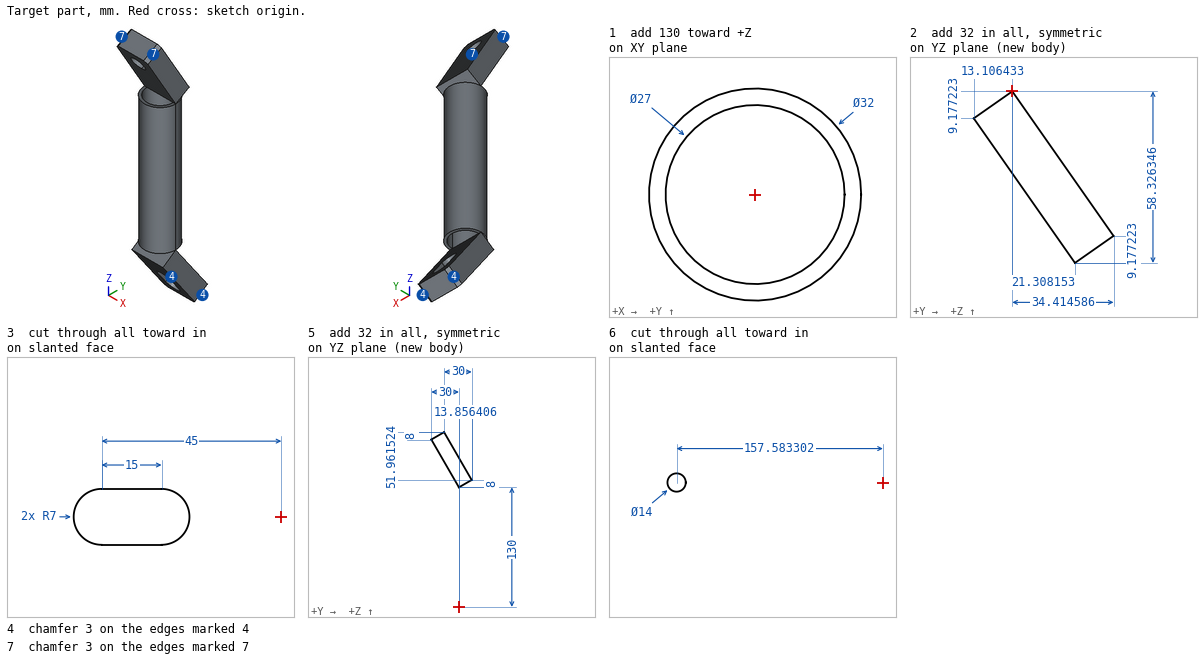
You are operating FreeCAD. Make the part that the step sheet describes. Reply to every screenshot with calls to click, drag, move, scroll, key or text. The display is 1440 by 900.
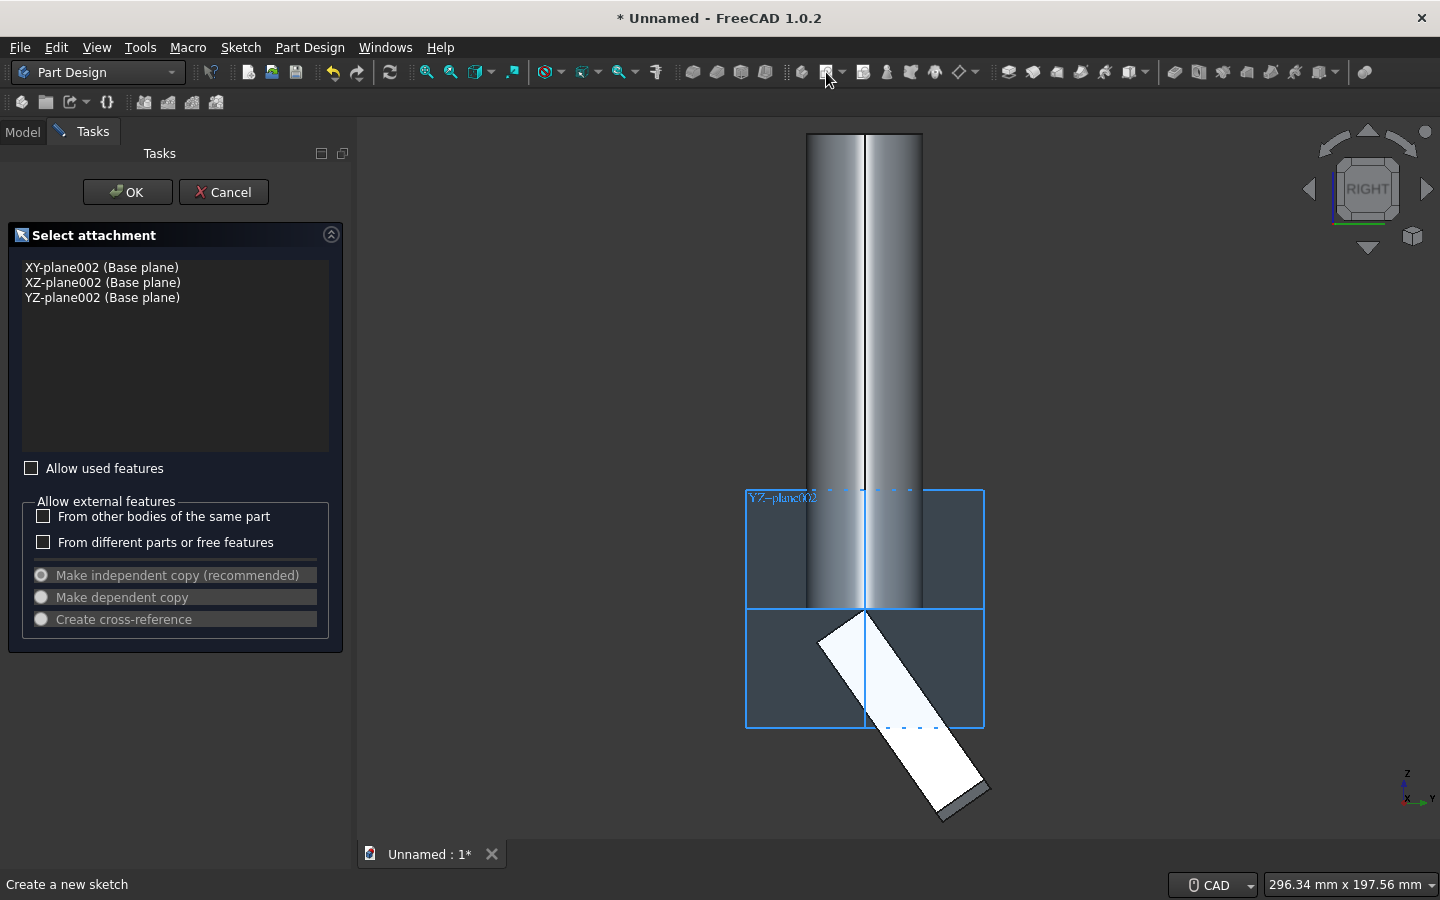
click(82, 298)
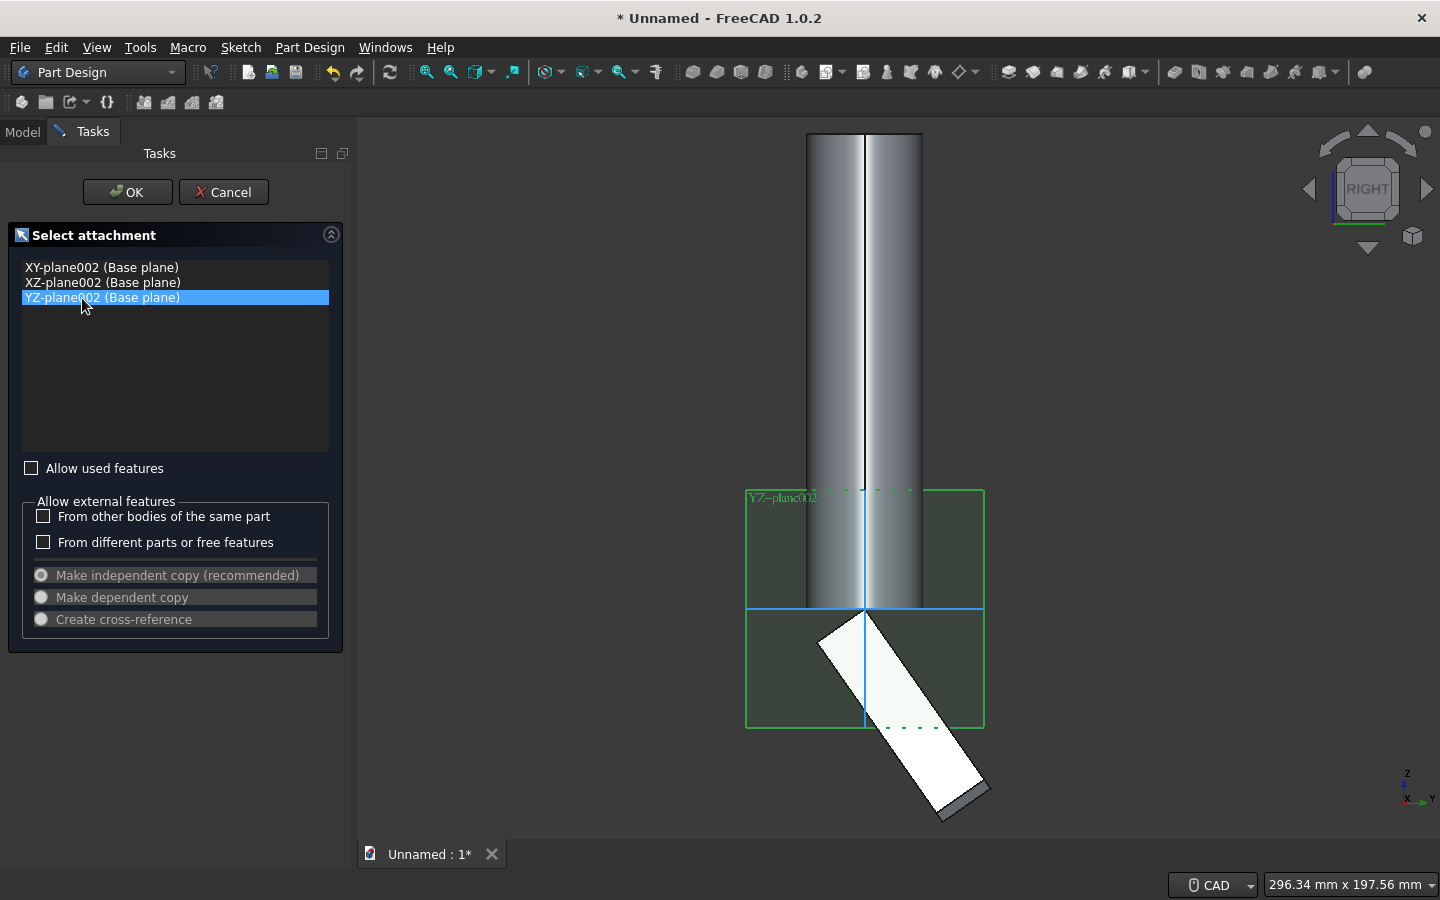
click(128, 192)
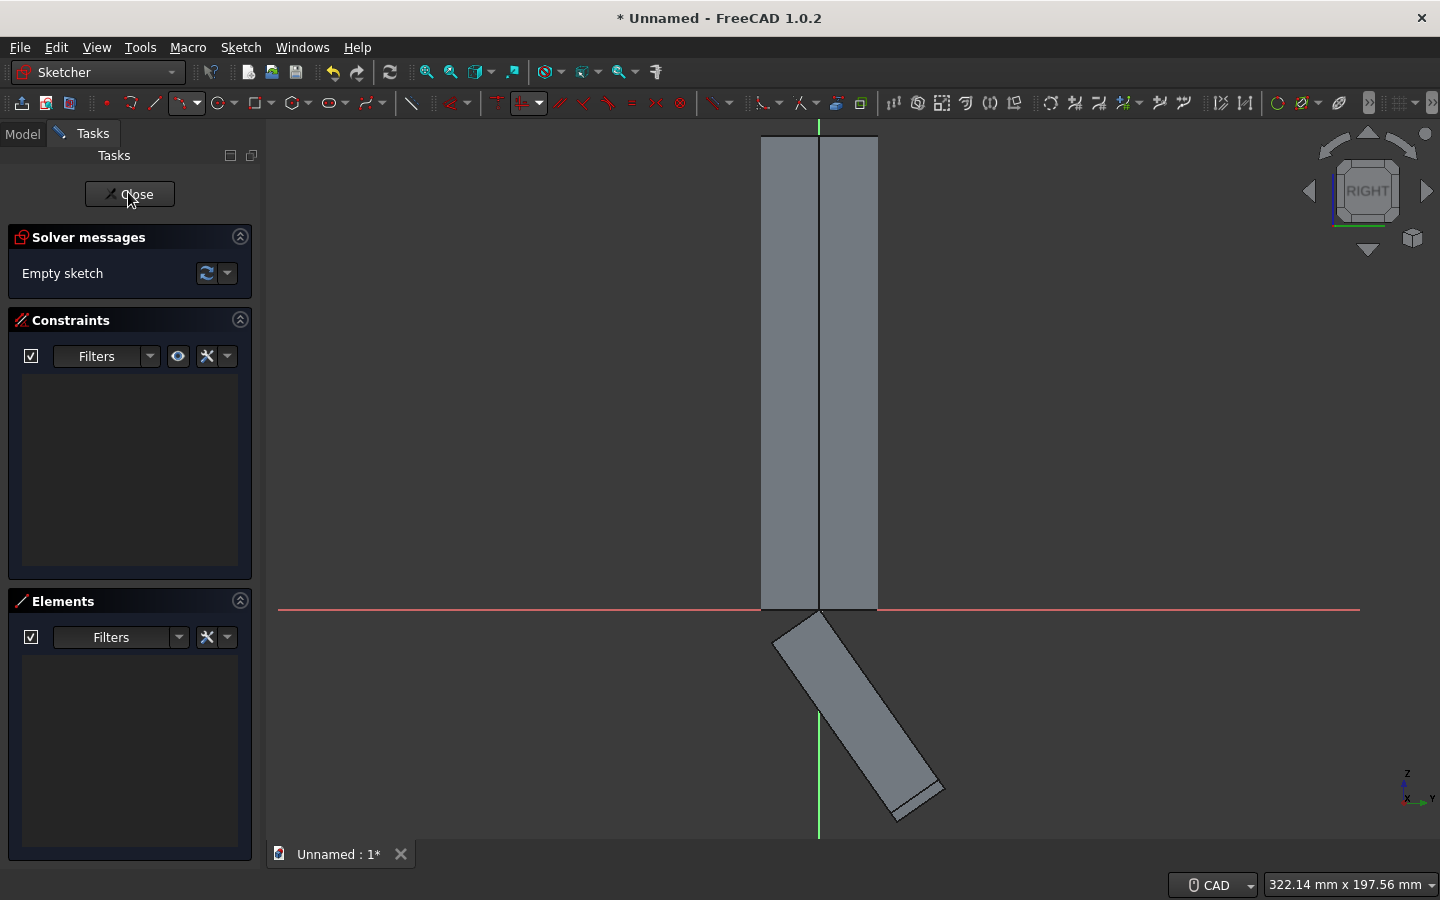
scroll(784, 479, down, 5)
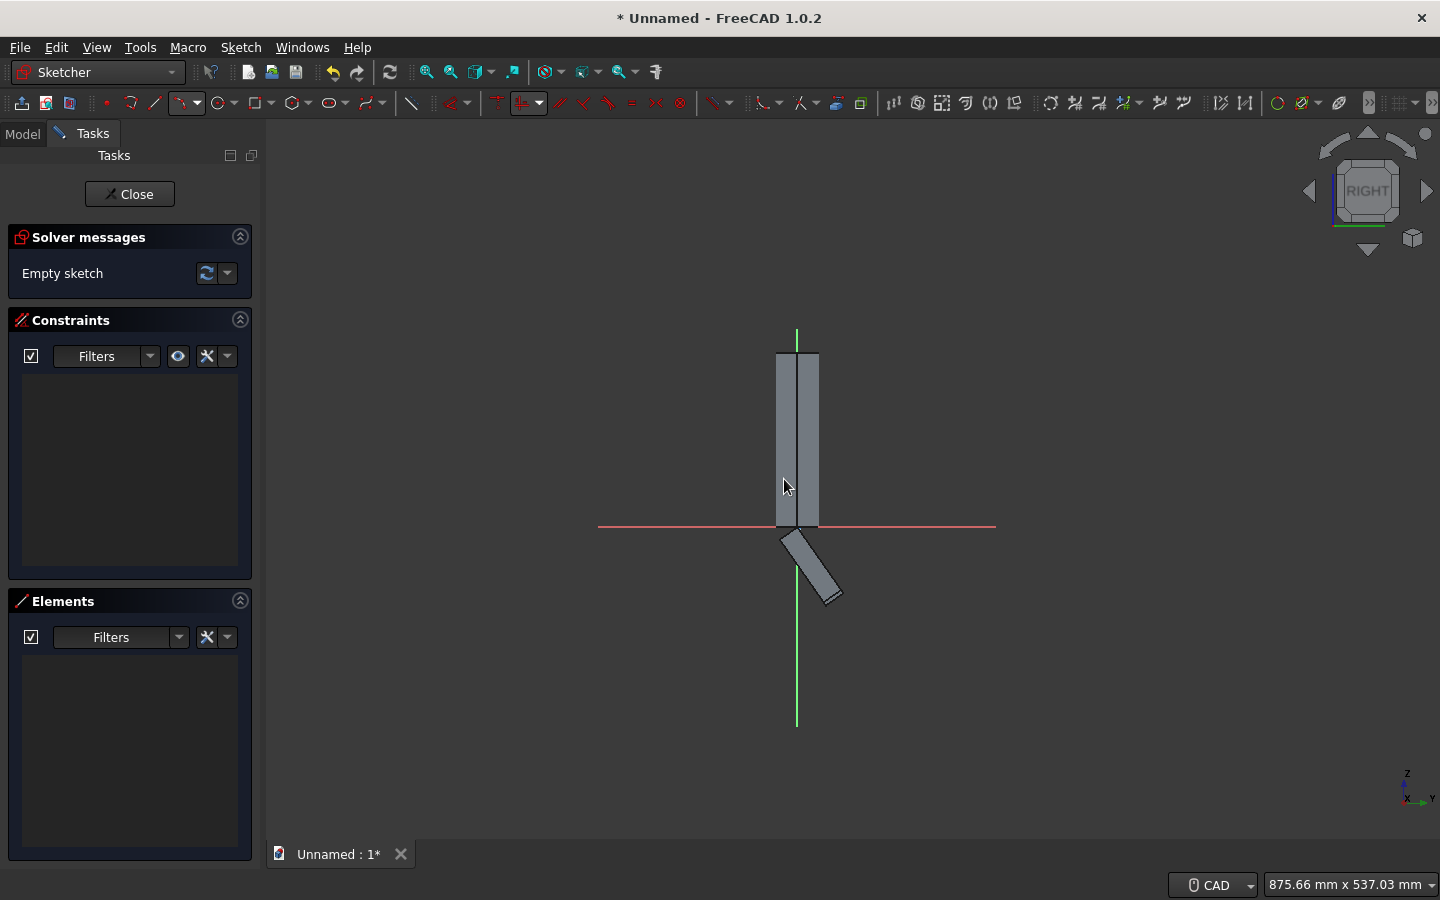
scroll(787, 280, up, 9)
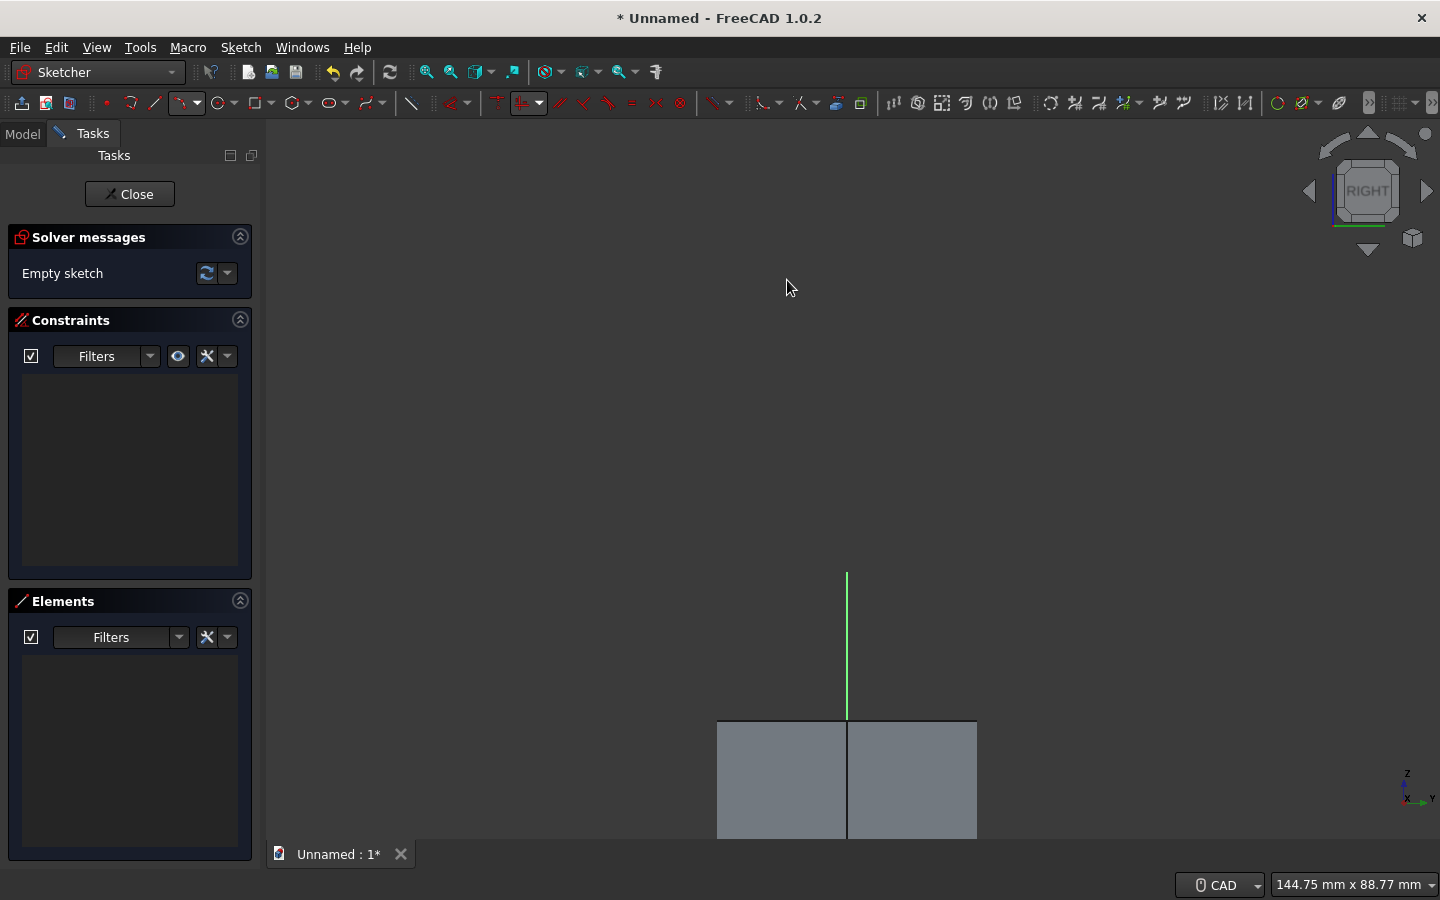
key(g)
key(m)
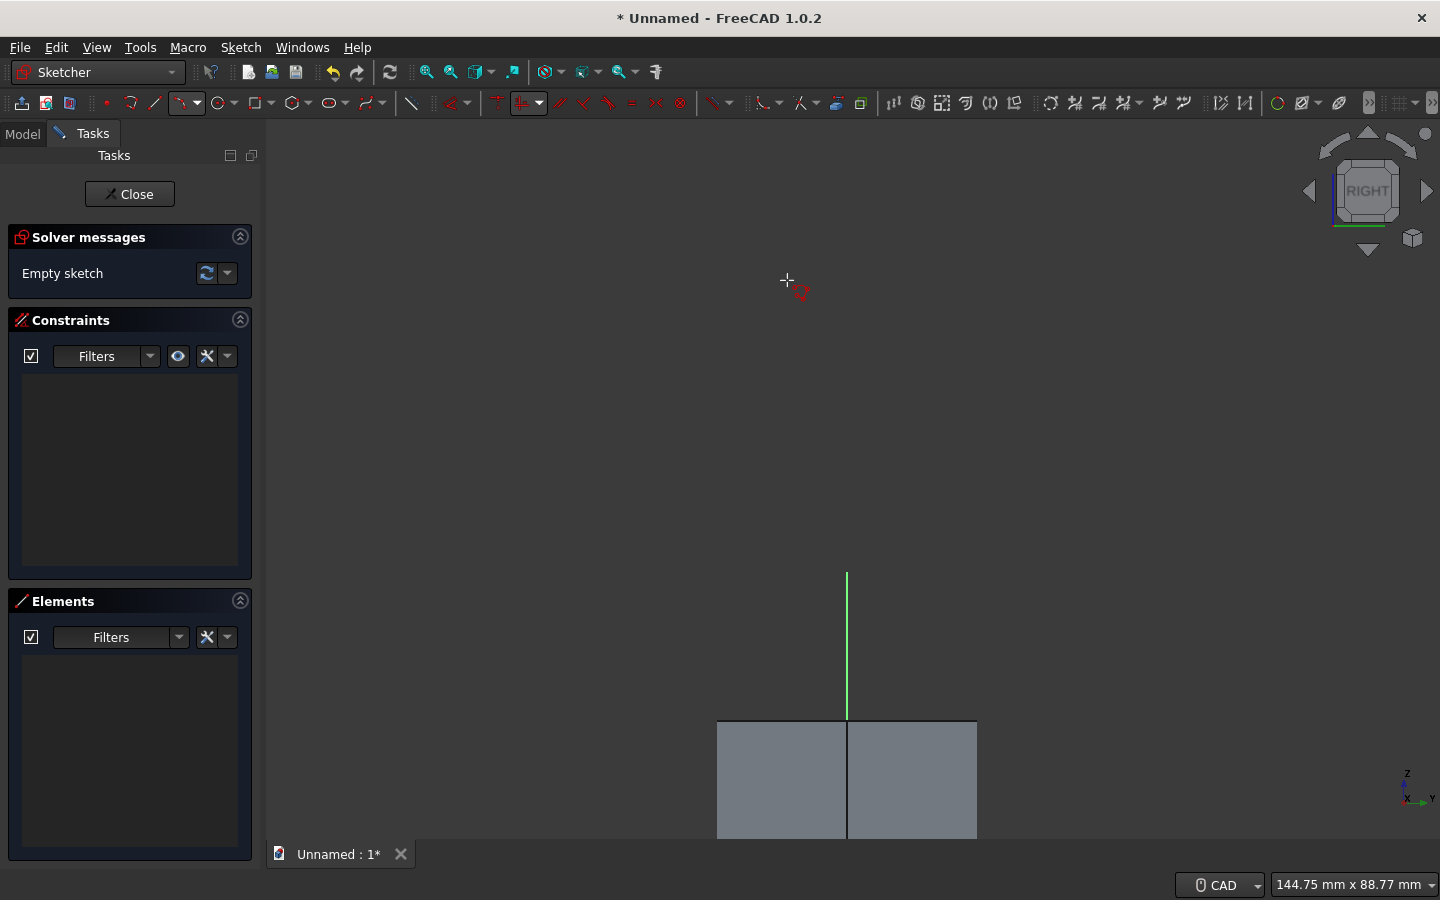
click(847, 721)
click(960, 656)
click(716, 235)
click(604, 299)
click(847, 722)
key(Escape)
key(Escape)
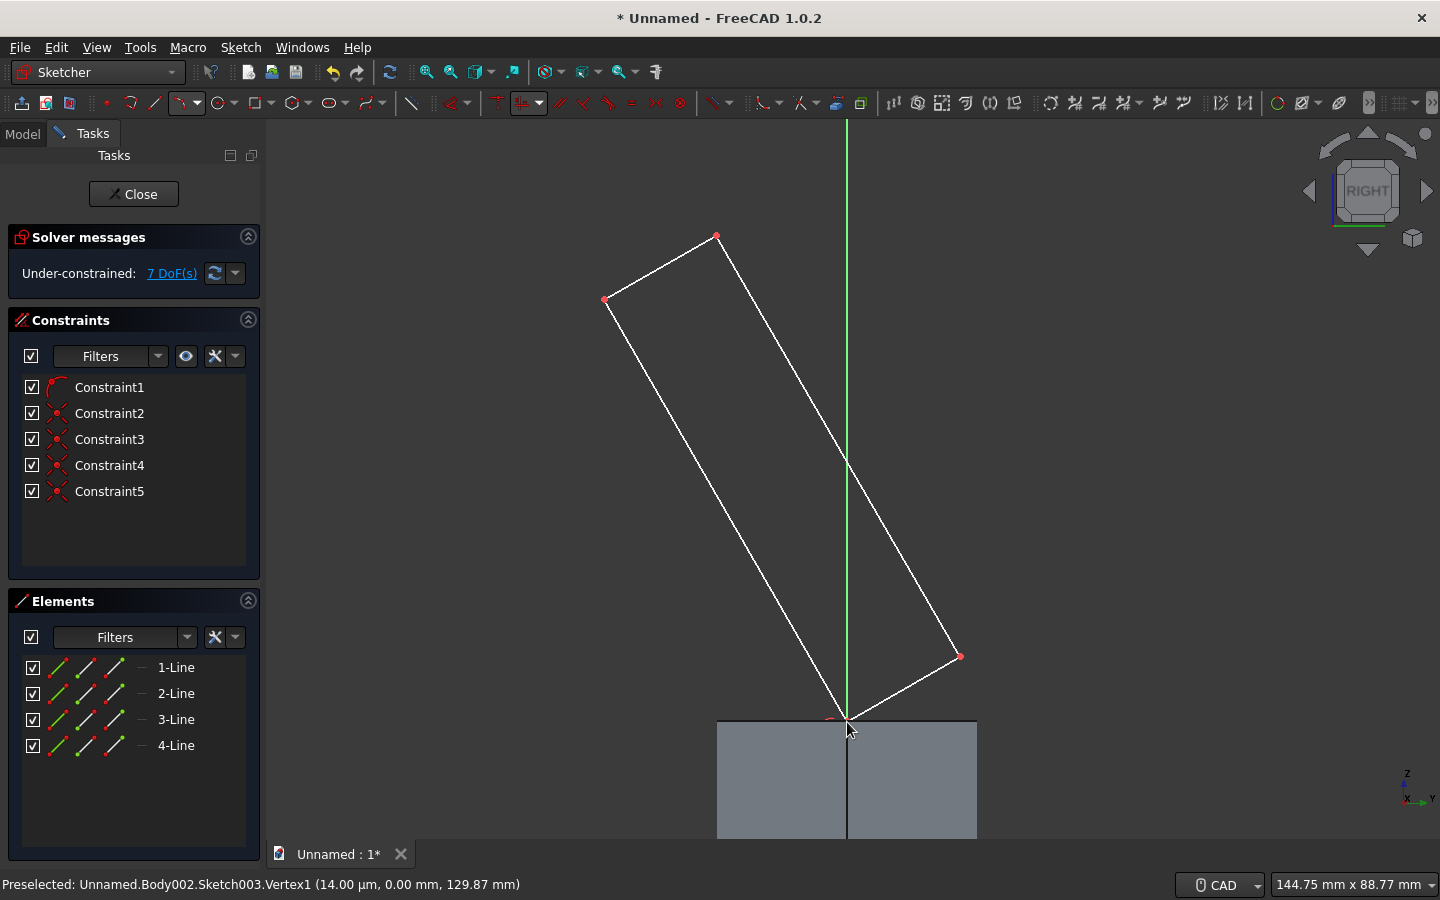
click(450, 104)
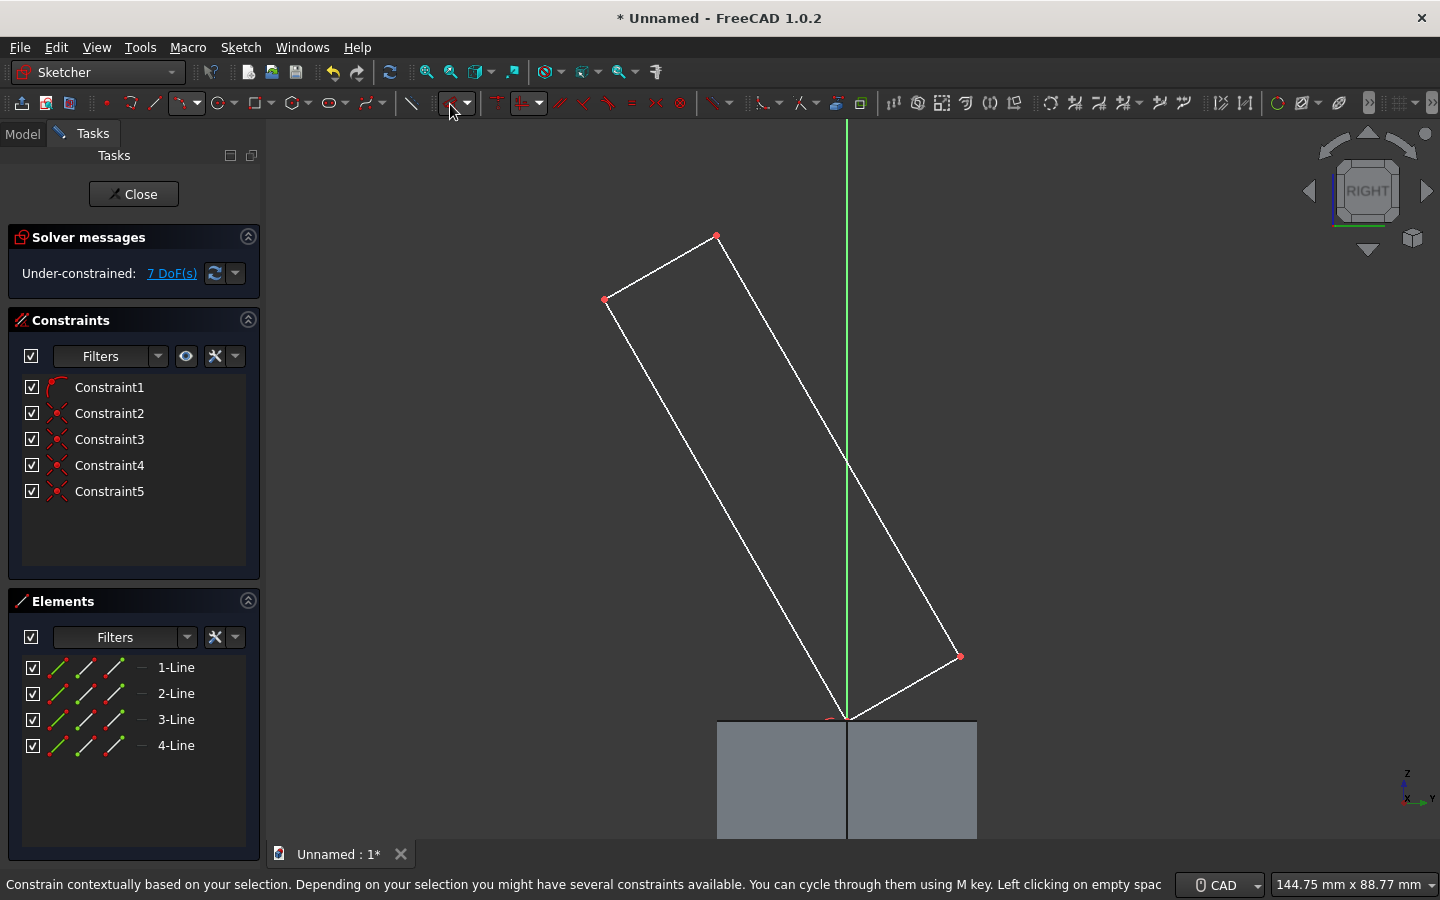
click(881, 703)
click(994, 690)